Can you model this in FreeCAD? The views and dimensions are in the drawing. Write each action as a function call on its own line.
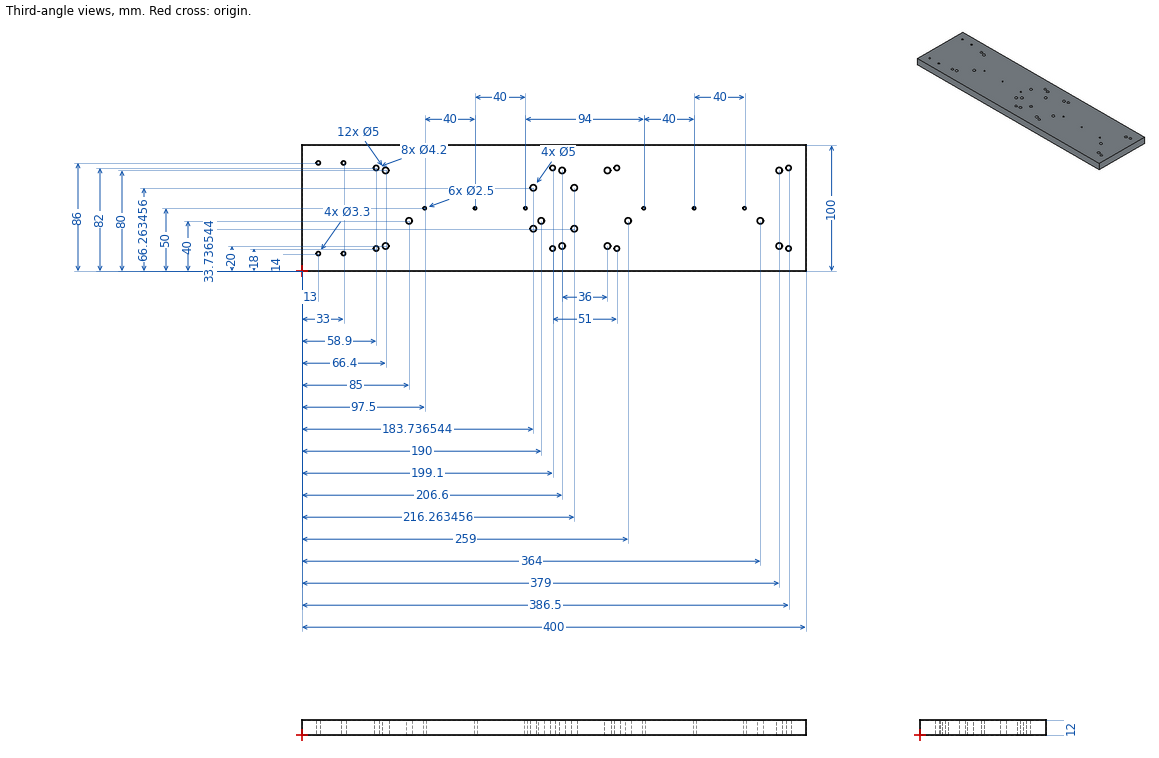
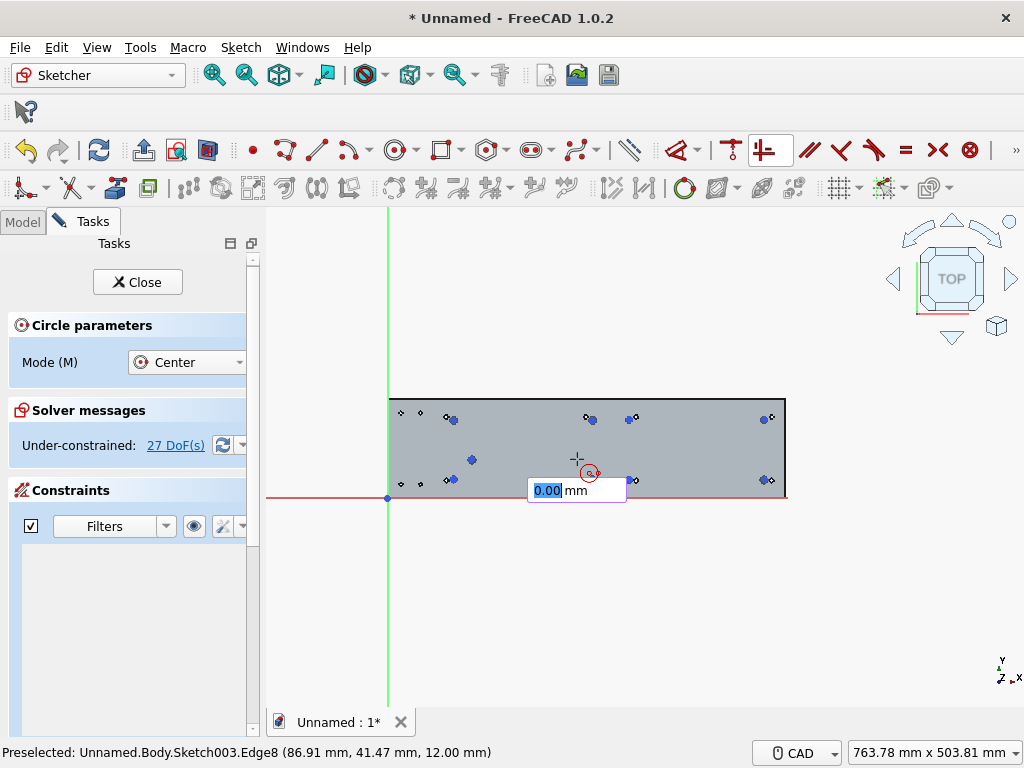
scroll(578, 457, up, 10)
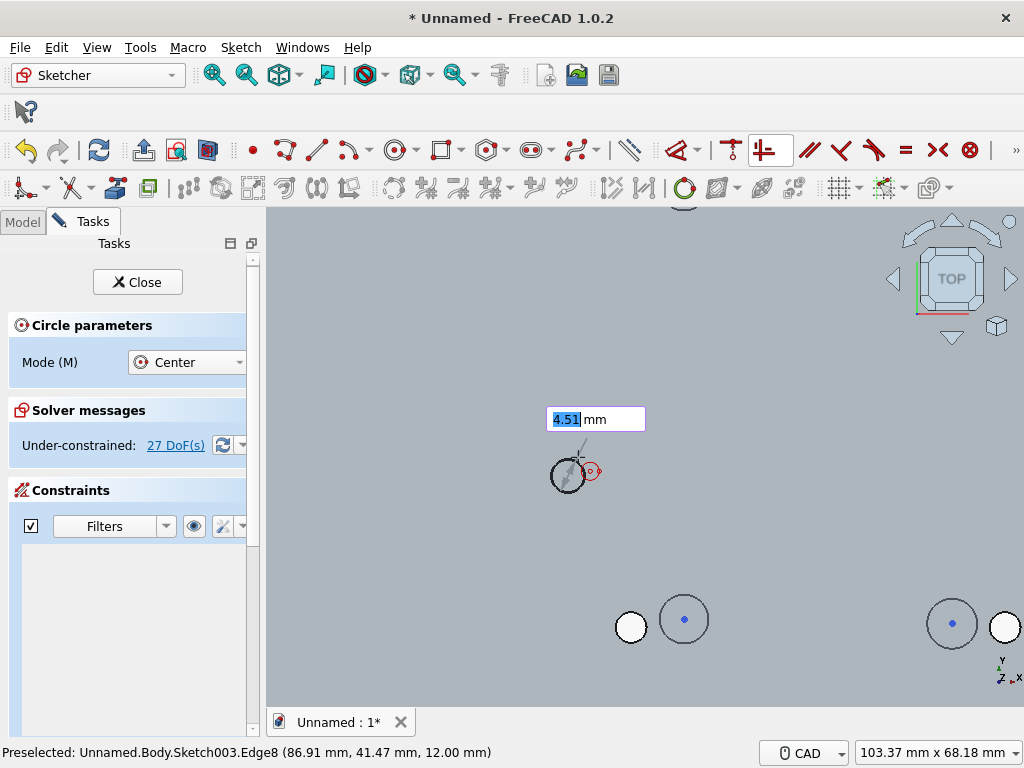
click(577, 453)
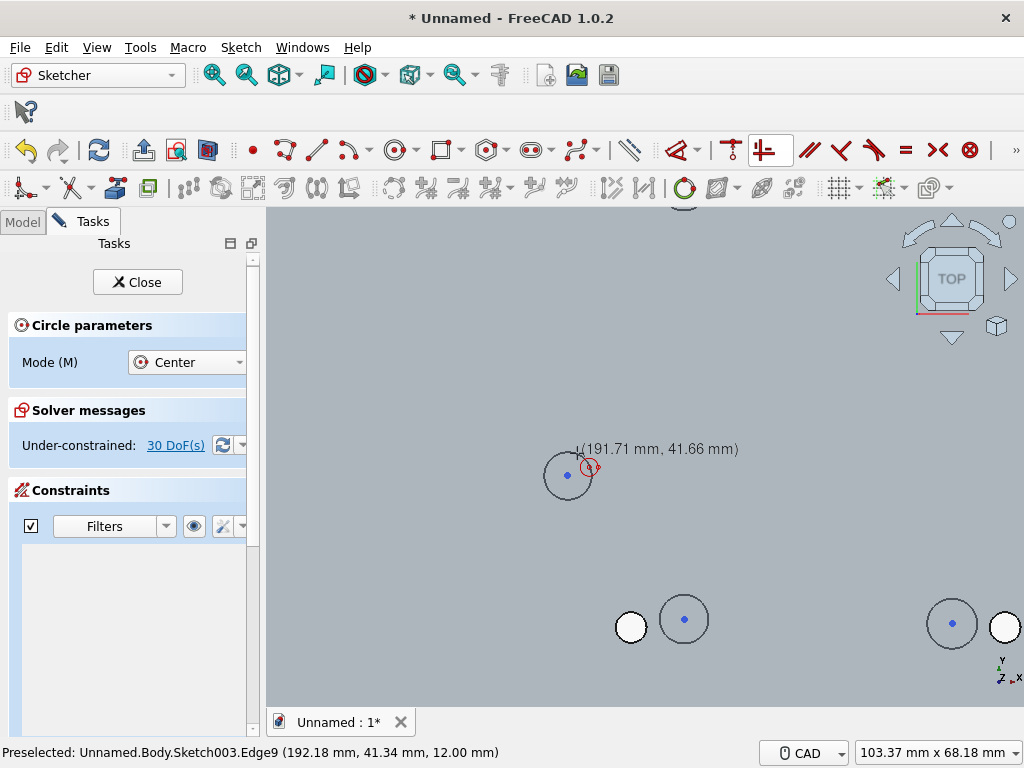
scroll(578, 457, down, 10)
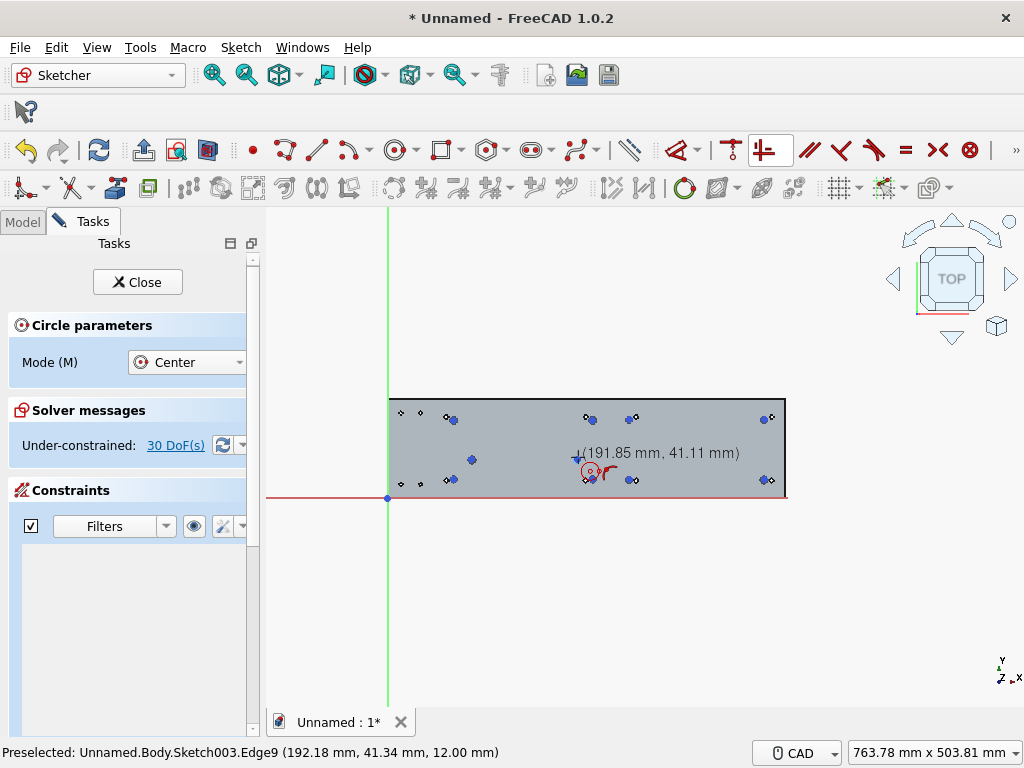
scroll(645, 459, up, 12)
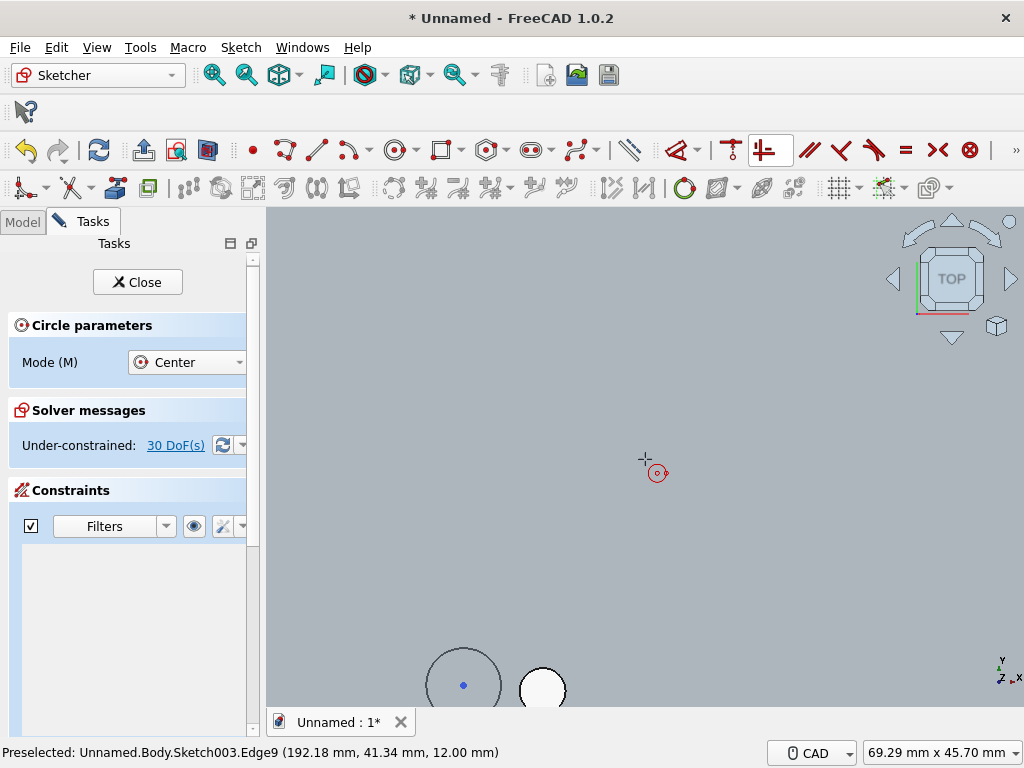
scroll(645, 459, down, 12)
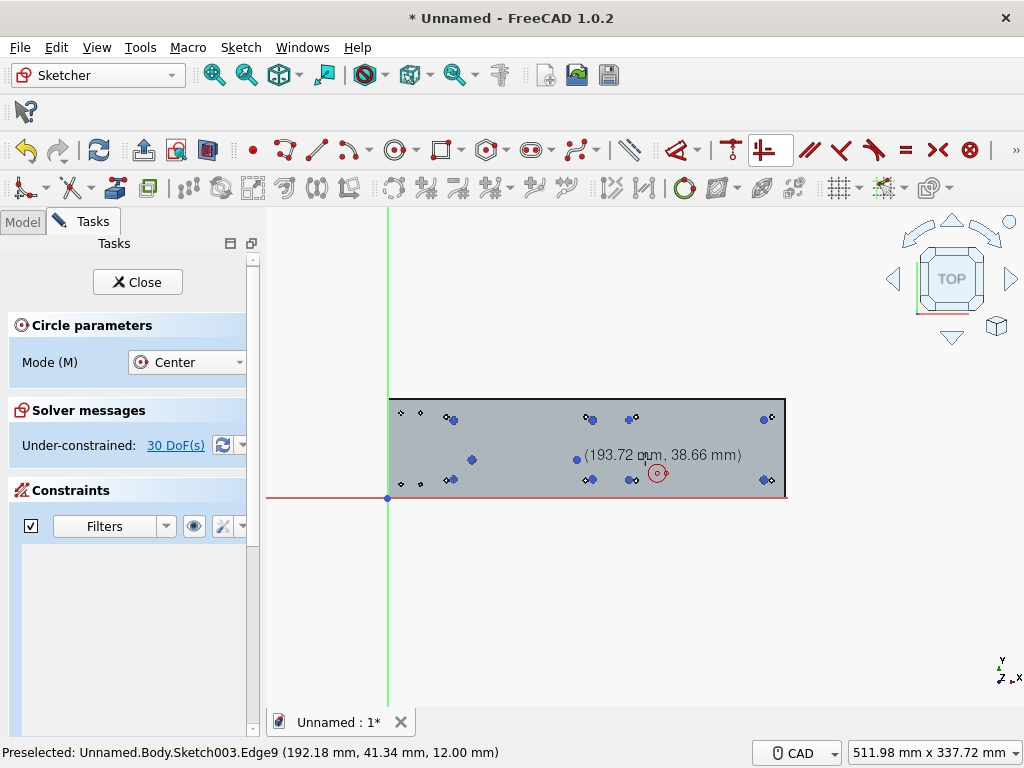
click(645, 459)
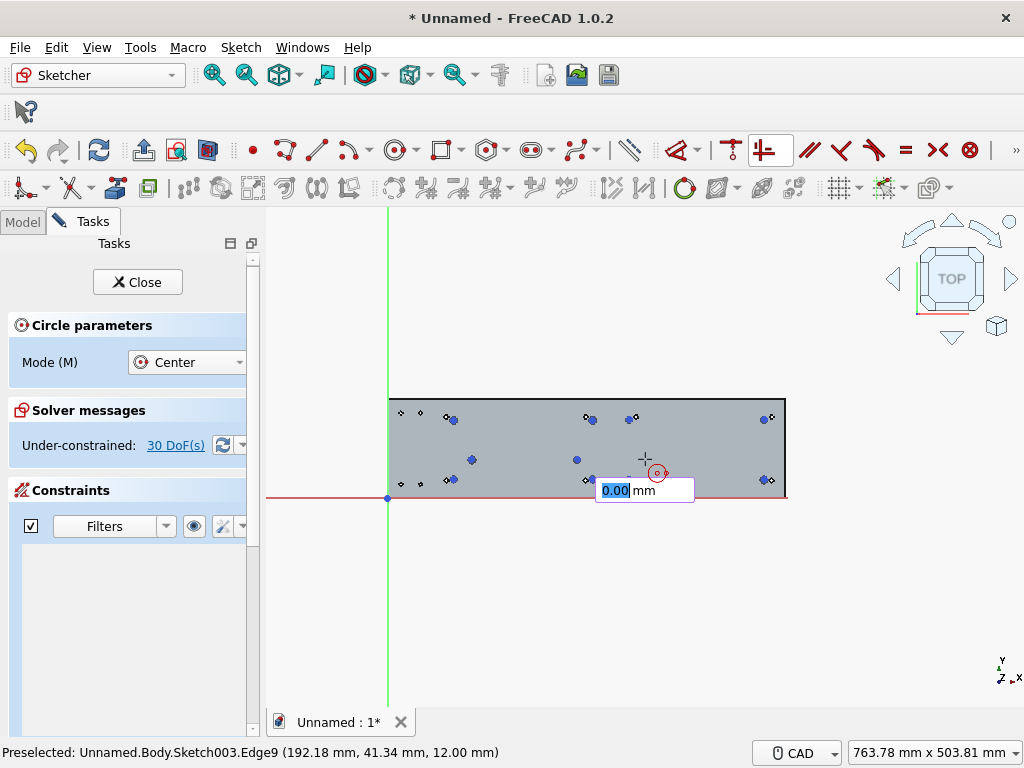
scroll(647, 457, up, 10)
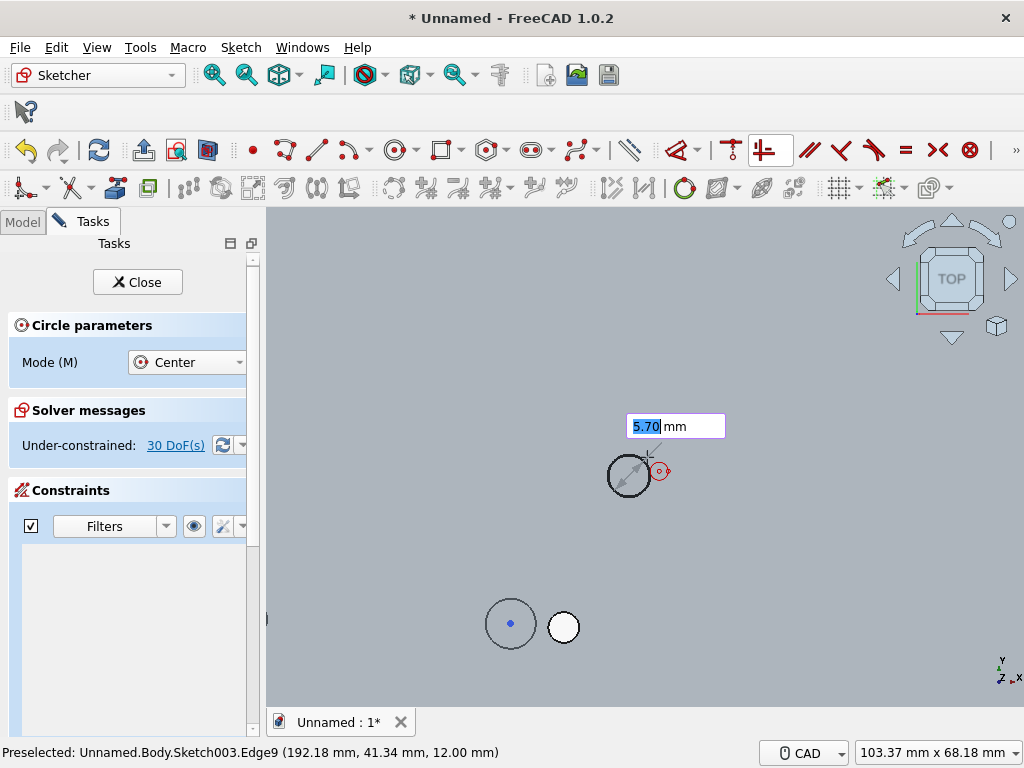
click(642, 453)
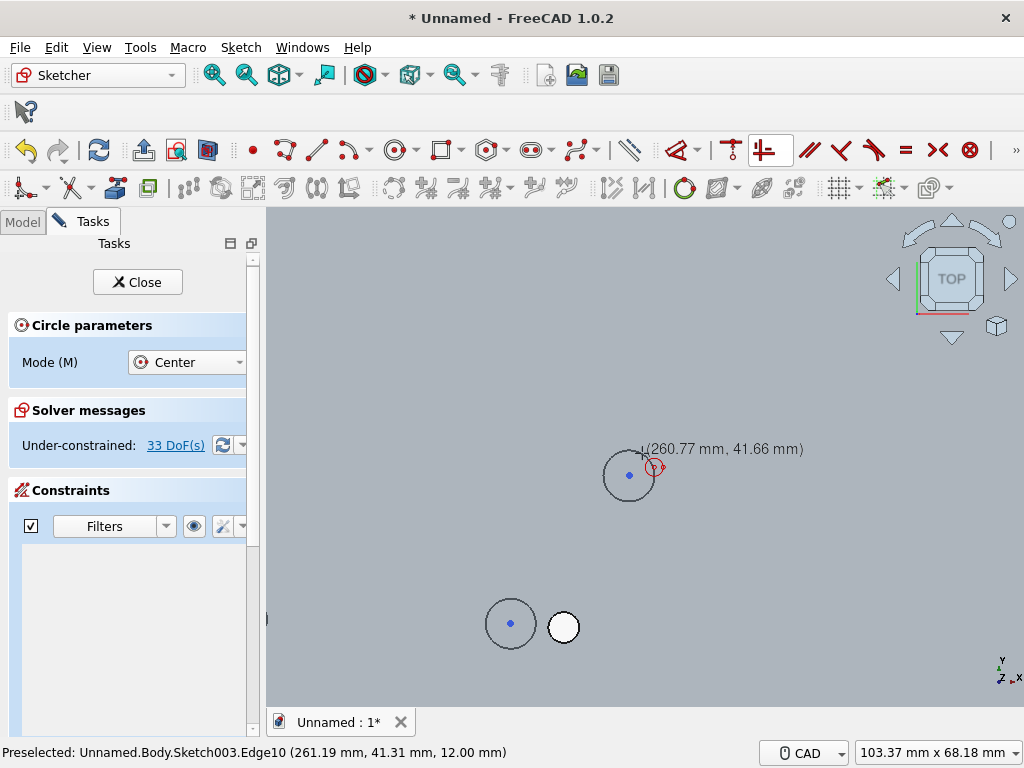
scroll(647, 457, down, 10)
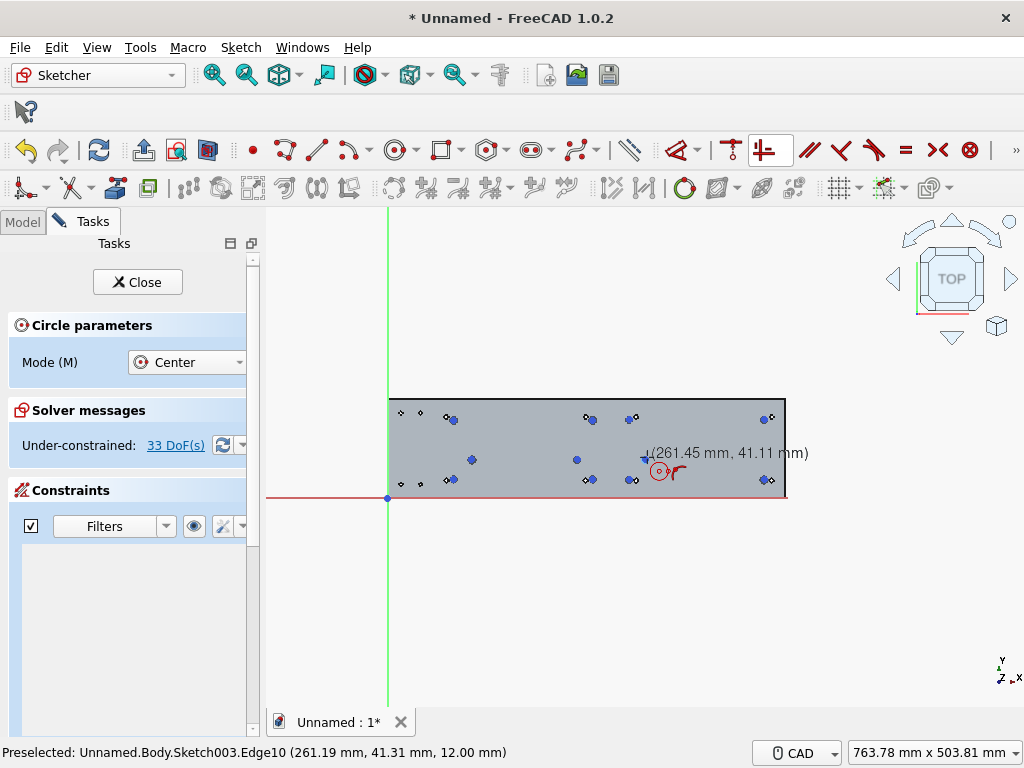
scroll(749, 459, up, 12)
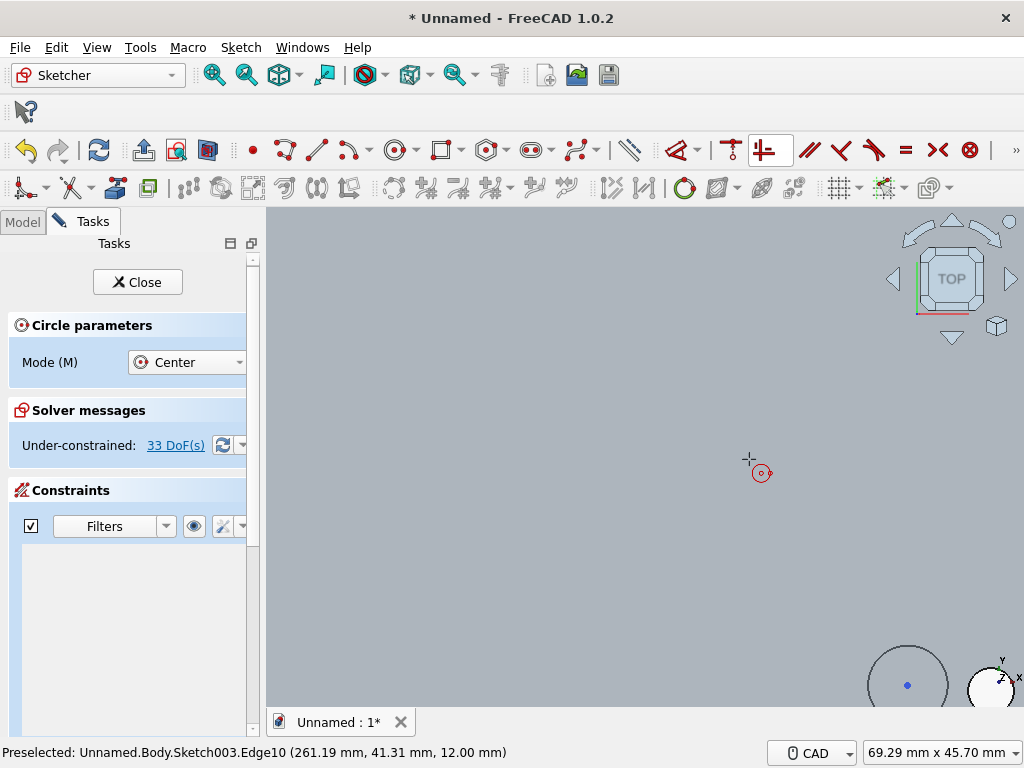
scroll(749, 459, down, 12)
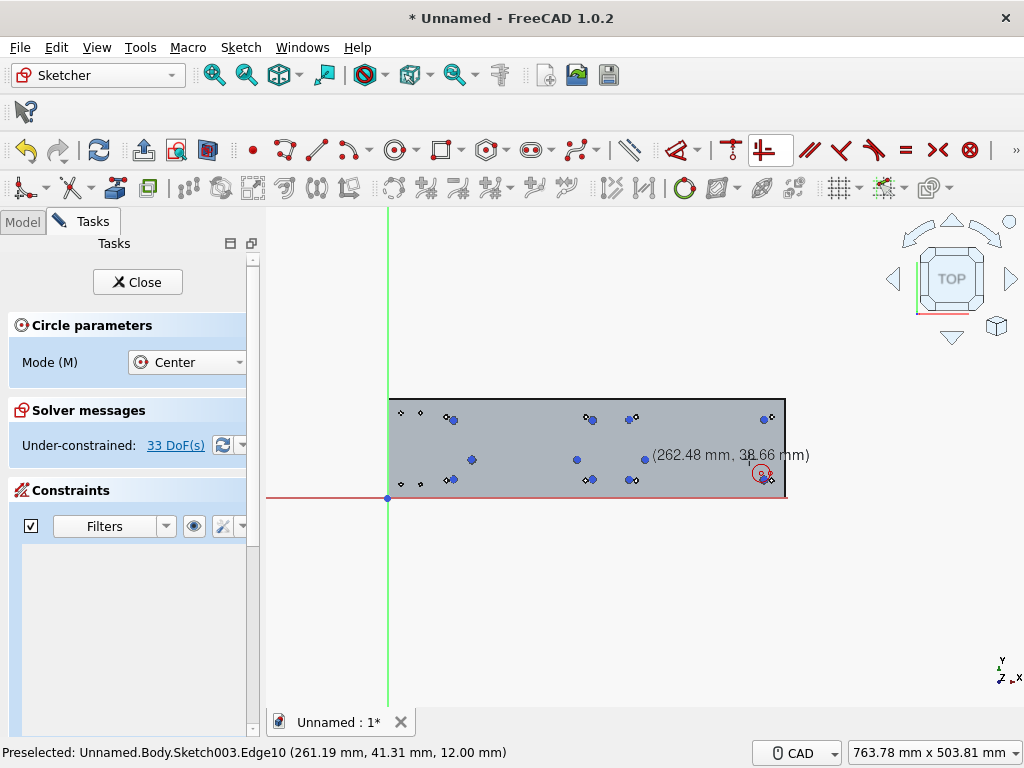
click(749, 459)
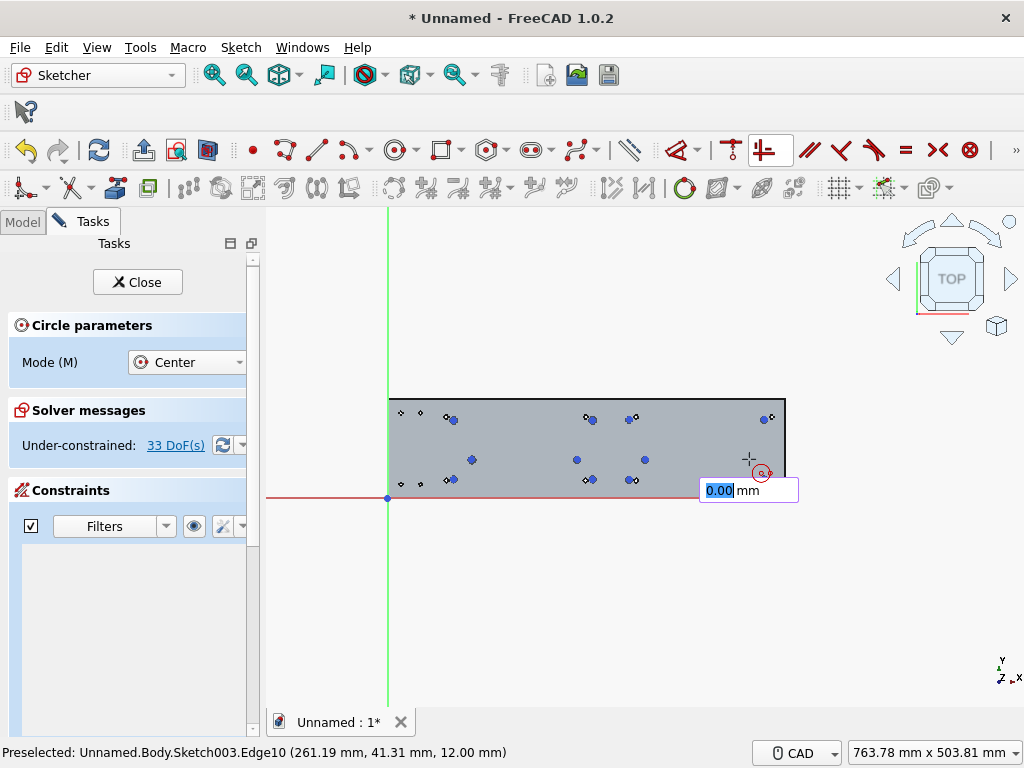
scroll(751, 457, up, 10)